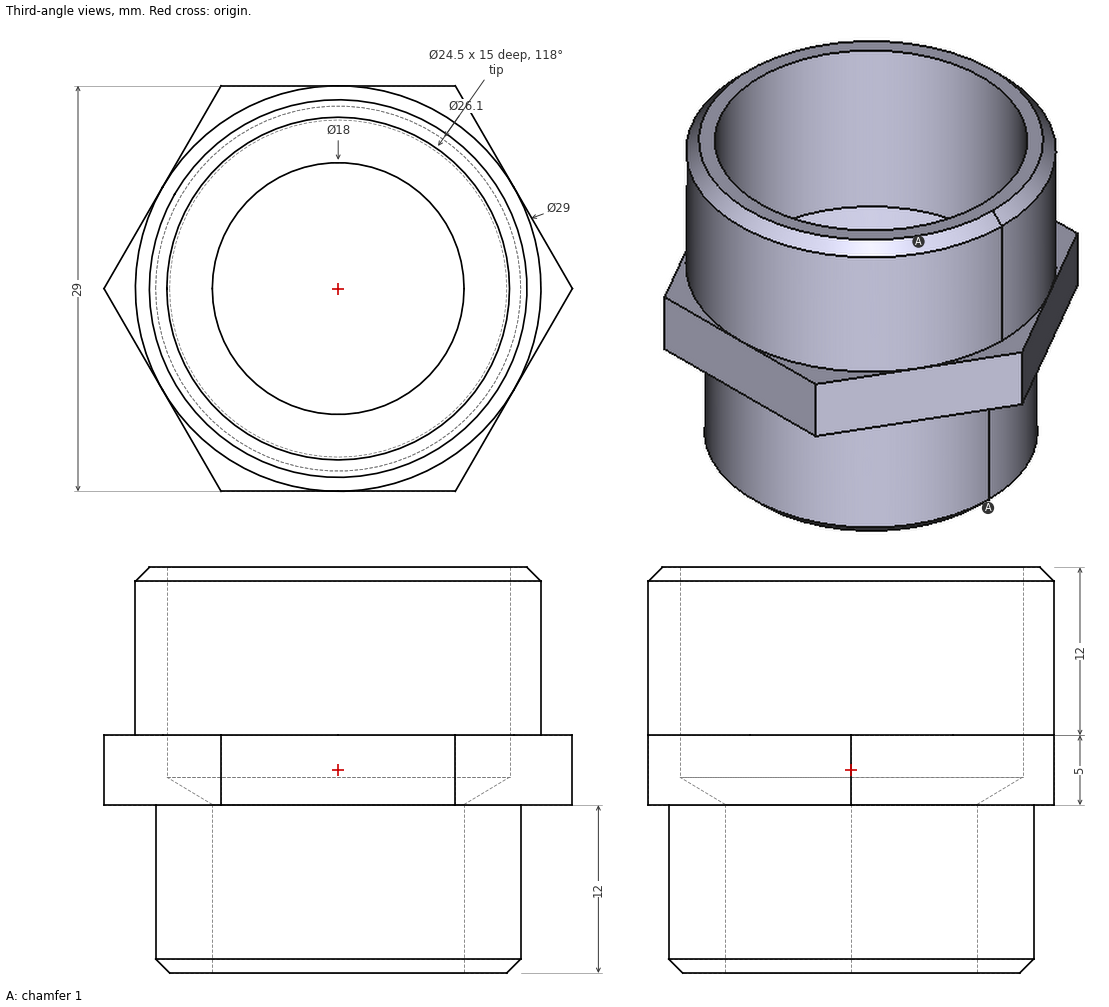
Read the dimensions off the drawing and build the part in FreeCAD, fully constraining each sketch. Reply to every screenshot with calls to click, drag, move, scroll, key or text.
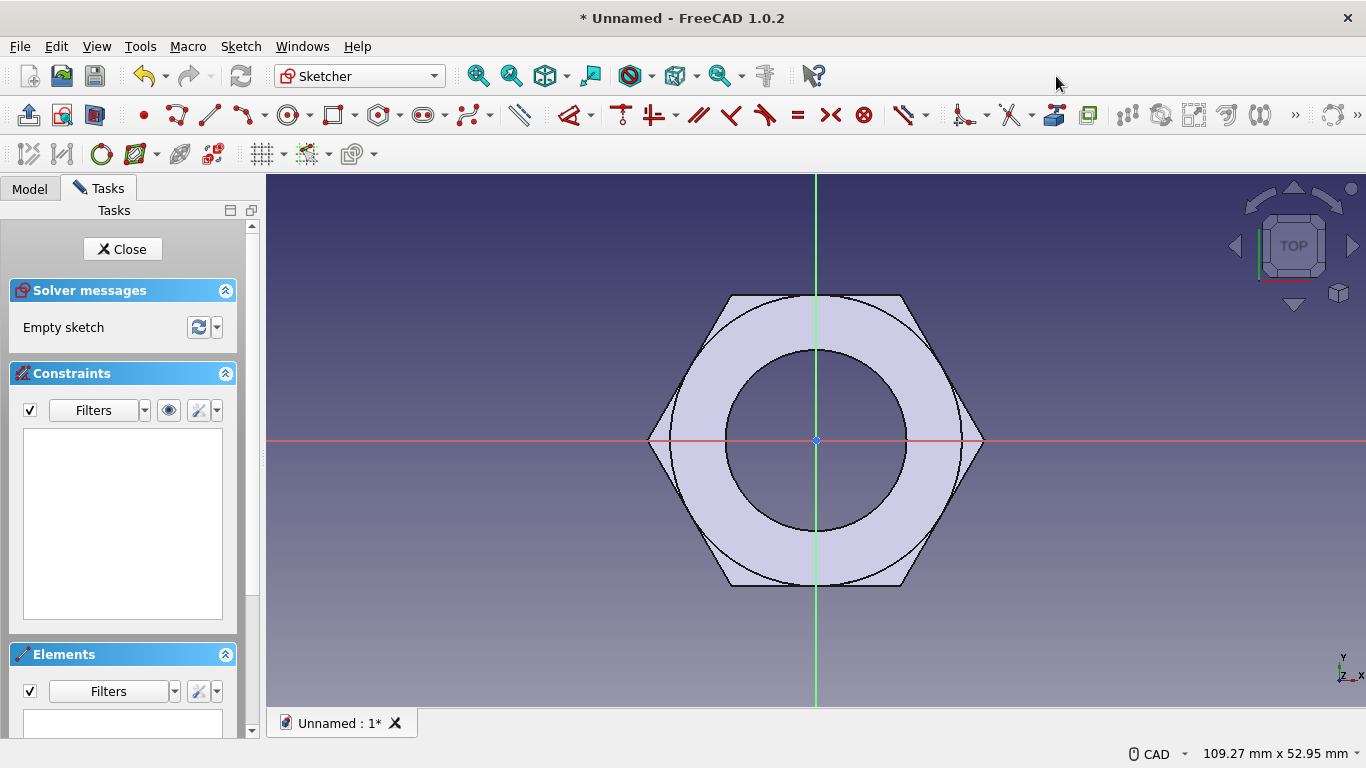
scroll(955, 440, up, 2)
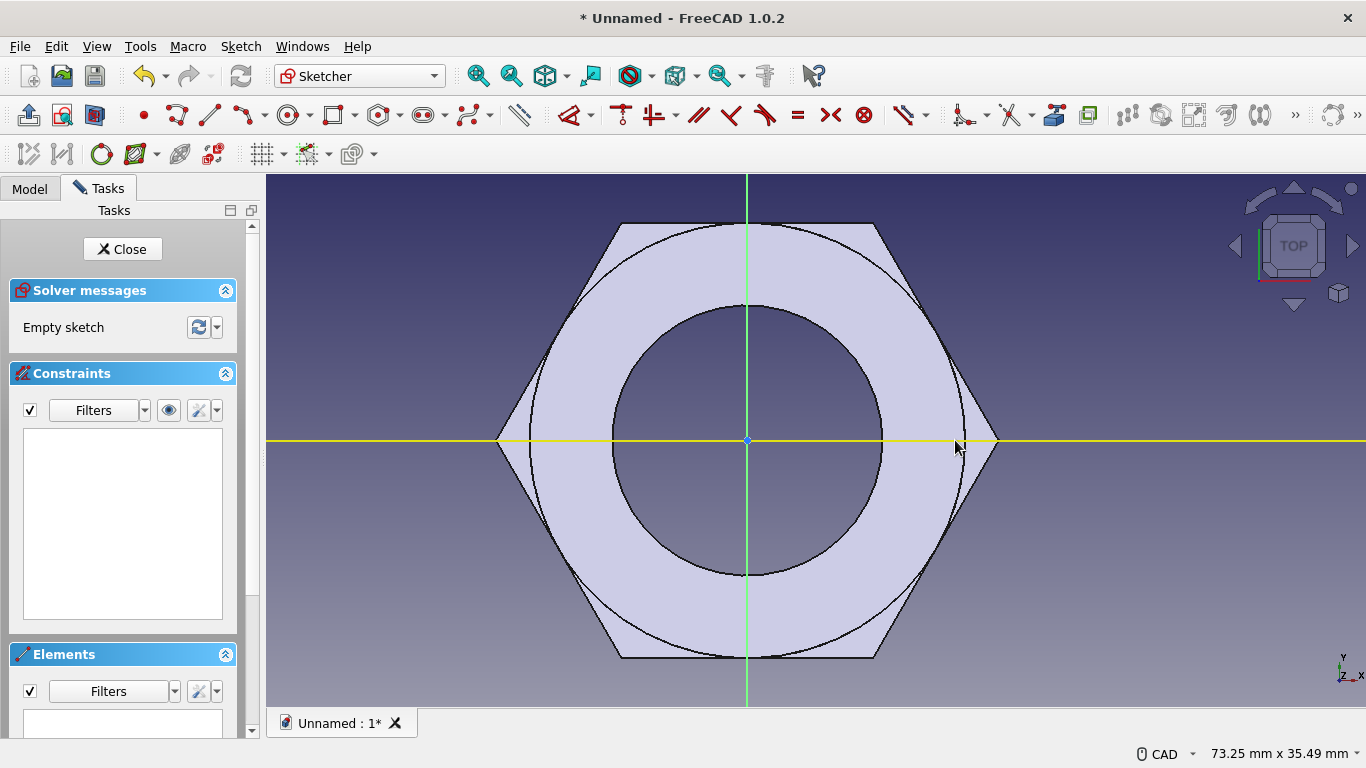
click(288, 116)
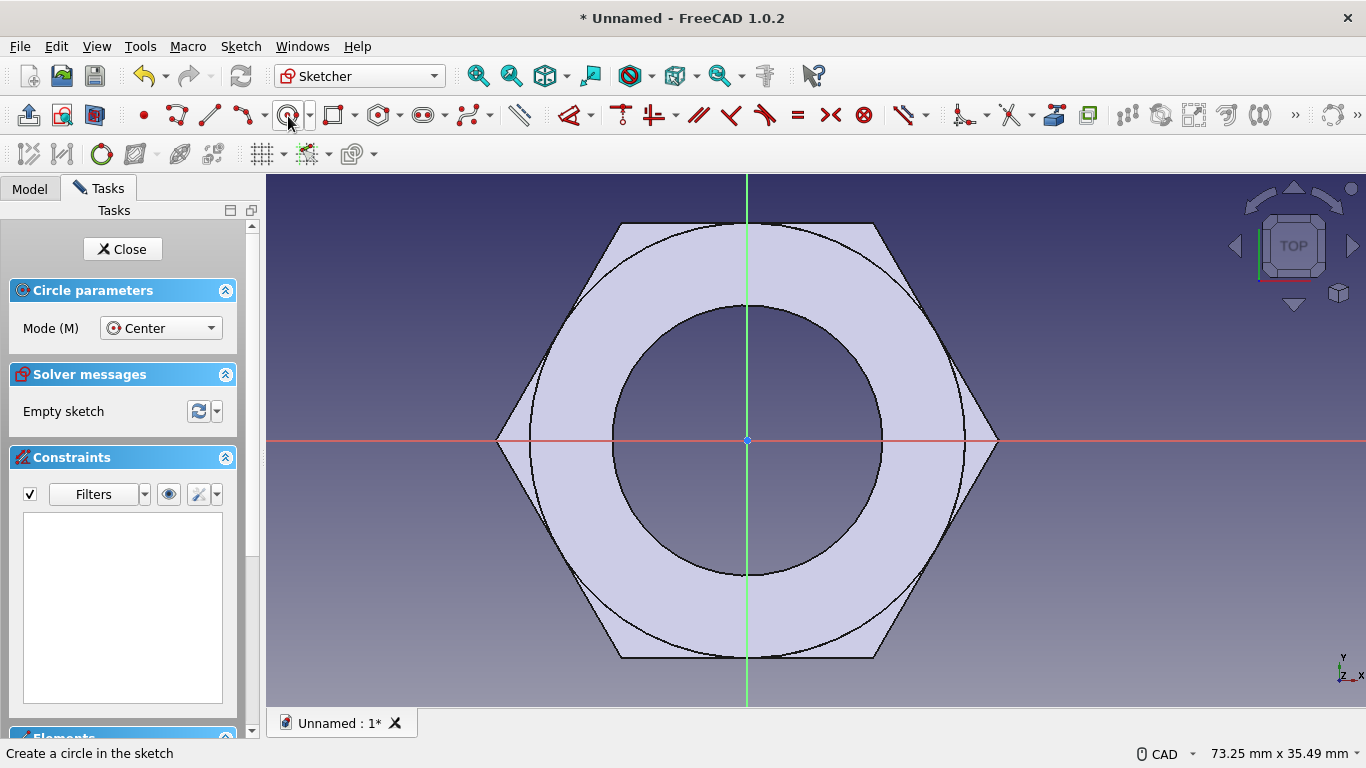
click(747, 440)
move(877, 310)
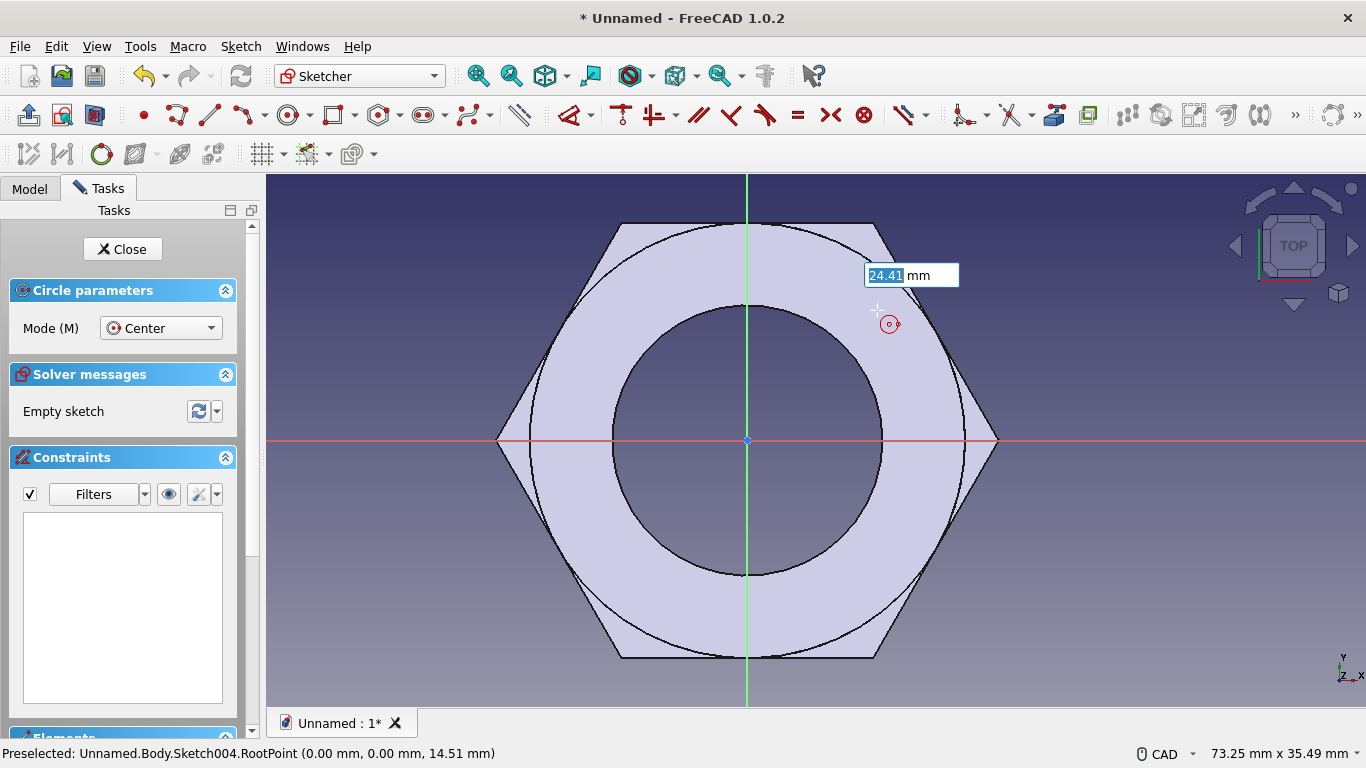
text(24.5)
key(Return)
key(Escape)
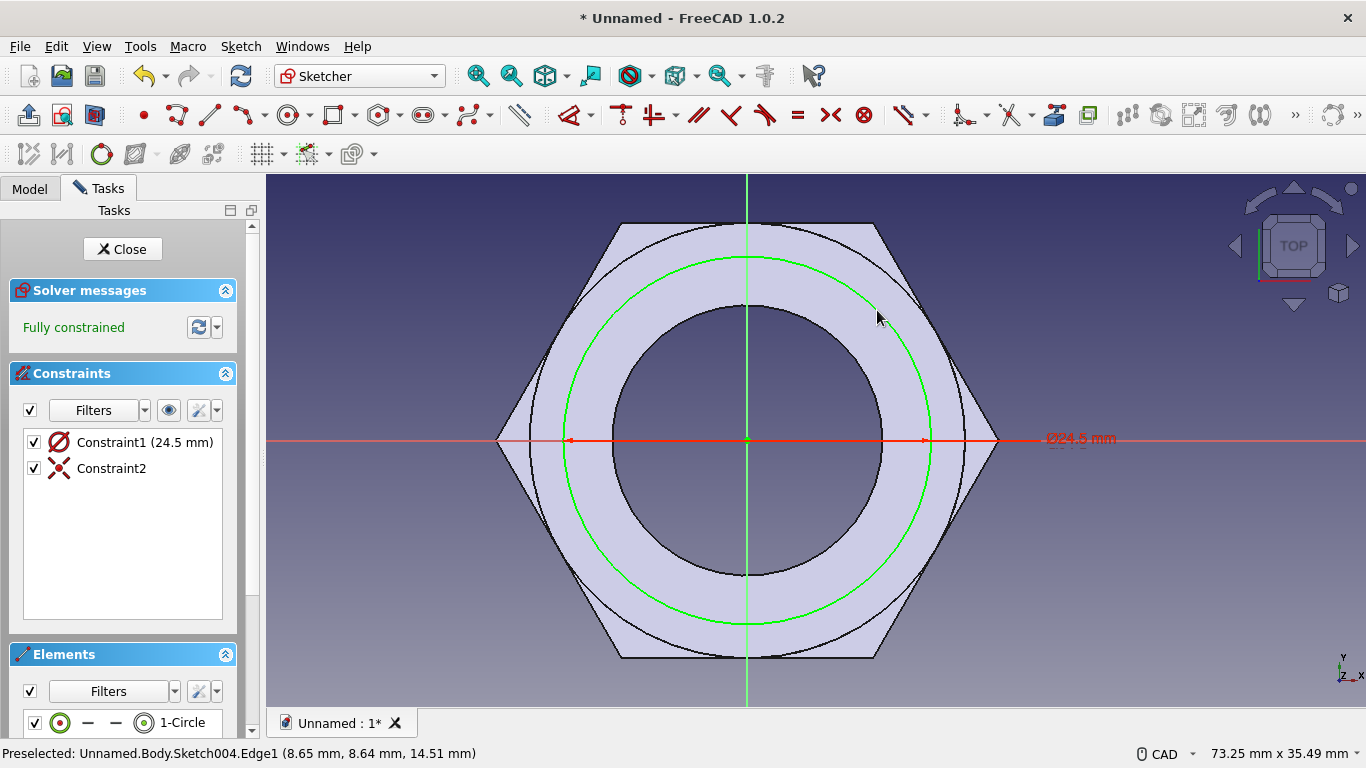
click(123, 249)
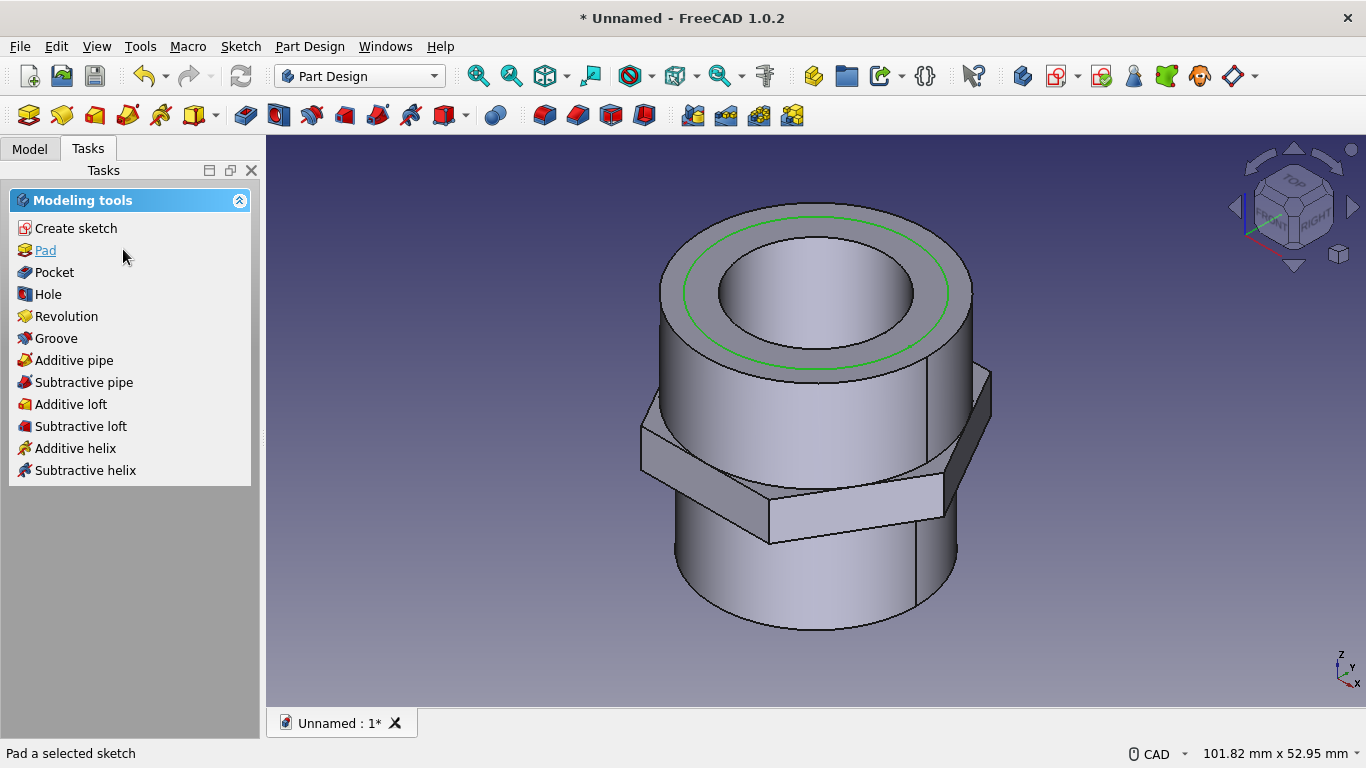
click(279, 116)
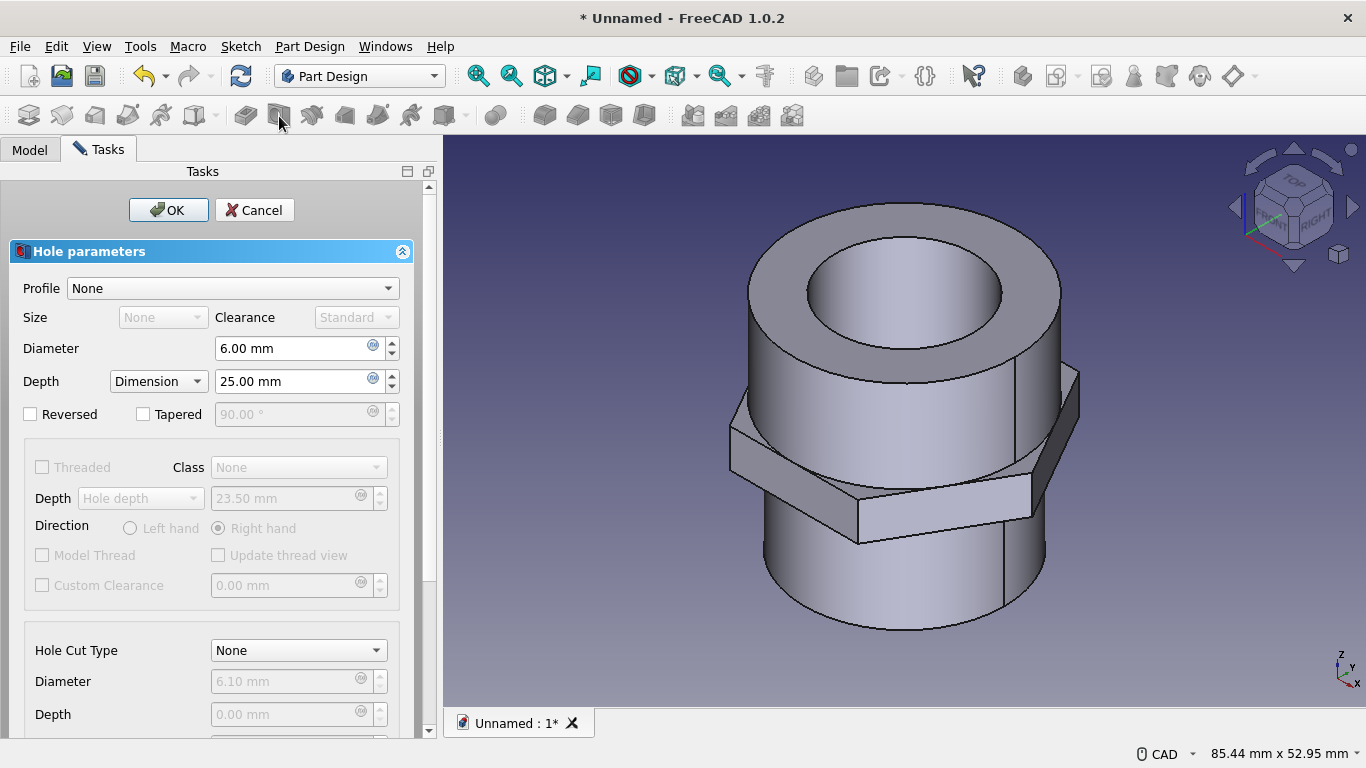
triple_click(300, 348)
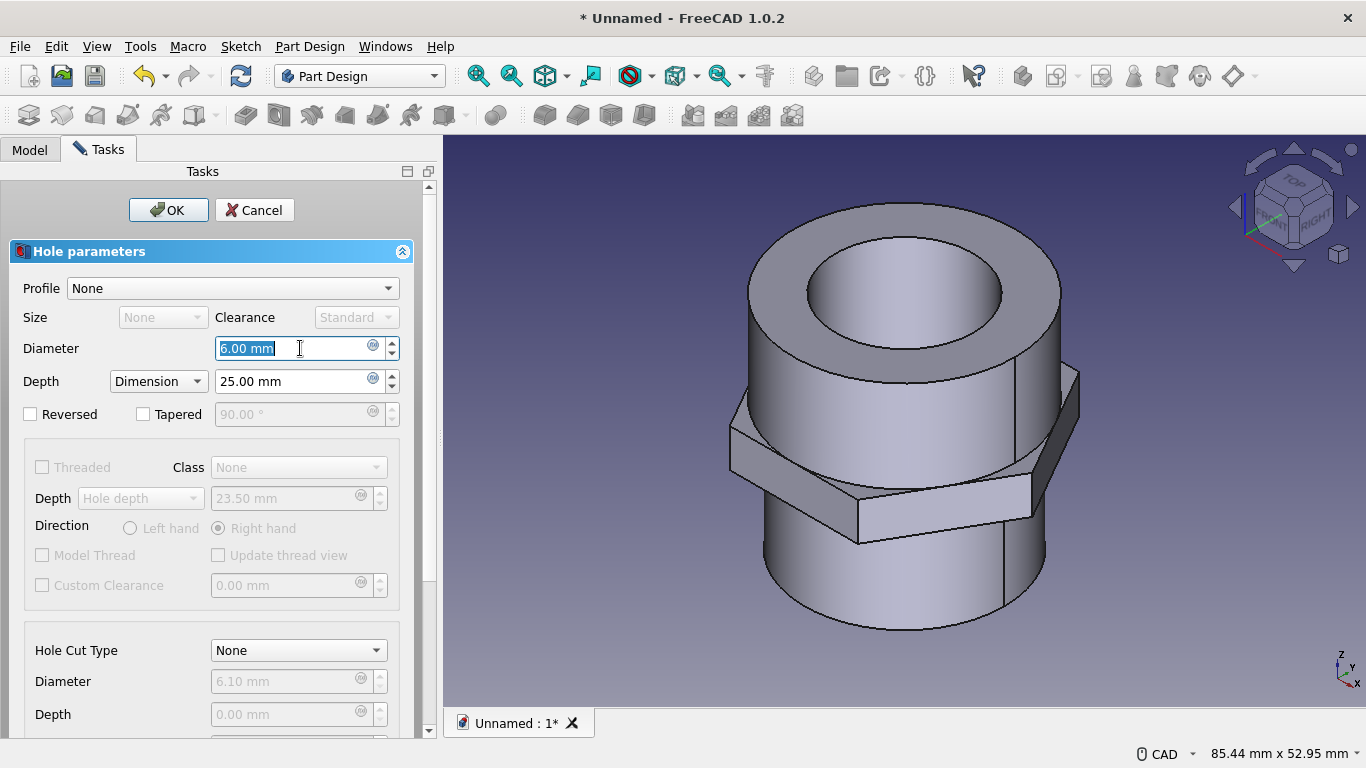
text(24.5)
key(Tab)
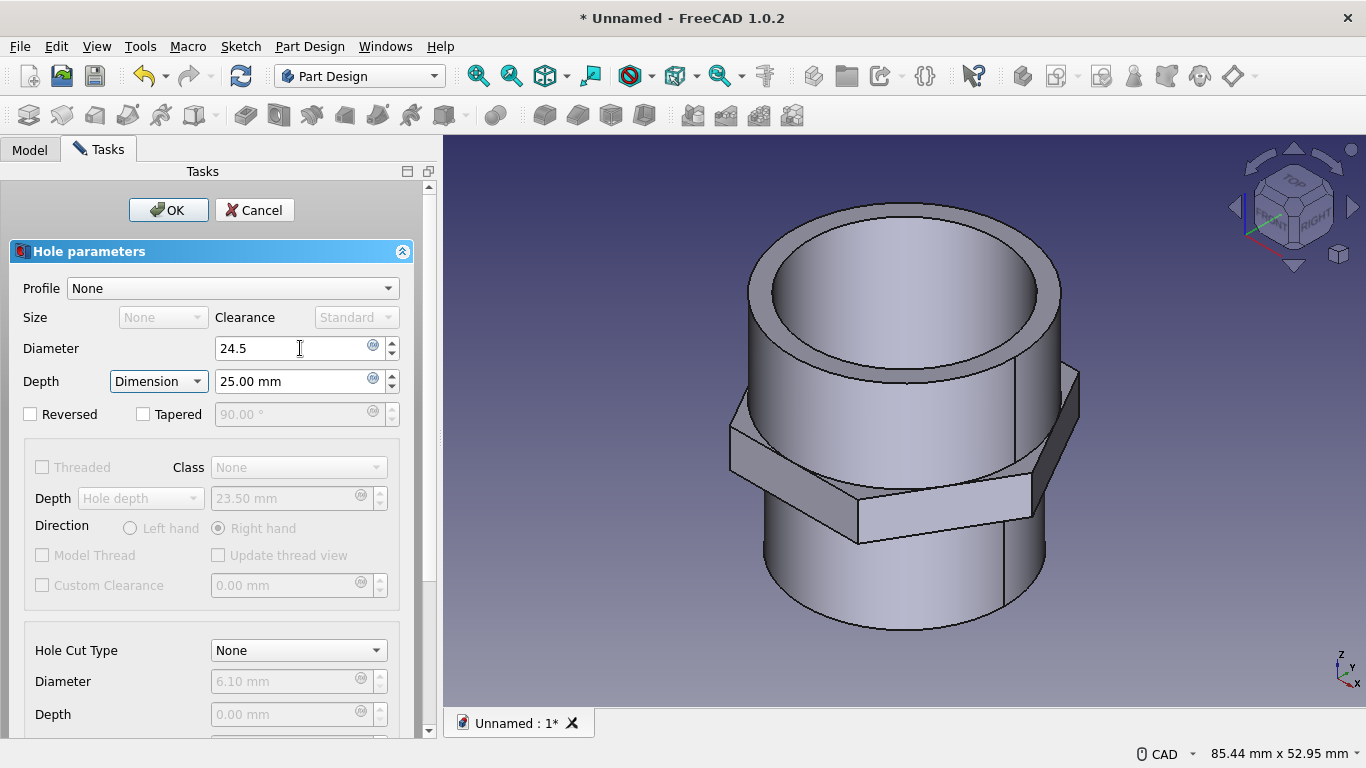
triple_click(300, 382)